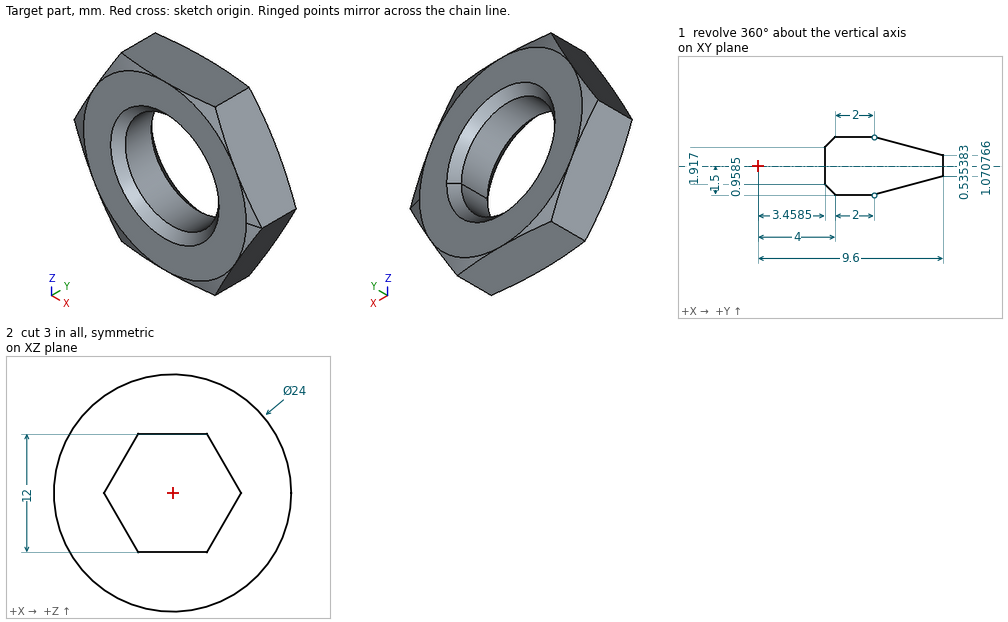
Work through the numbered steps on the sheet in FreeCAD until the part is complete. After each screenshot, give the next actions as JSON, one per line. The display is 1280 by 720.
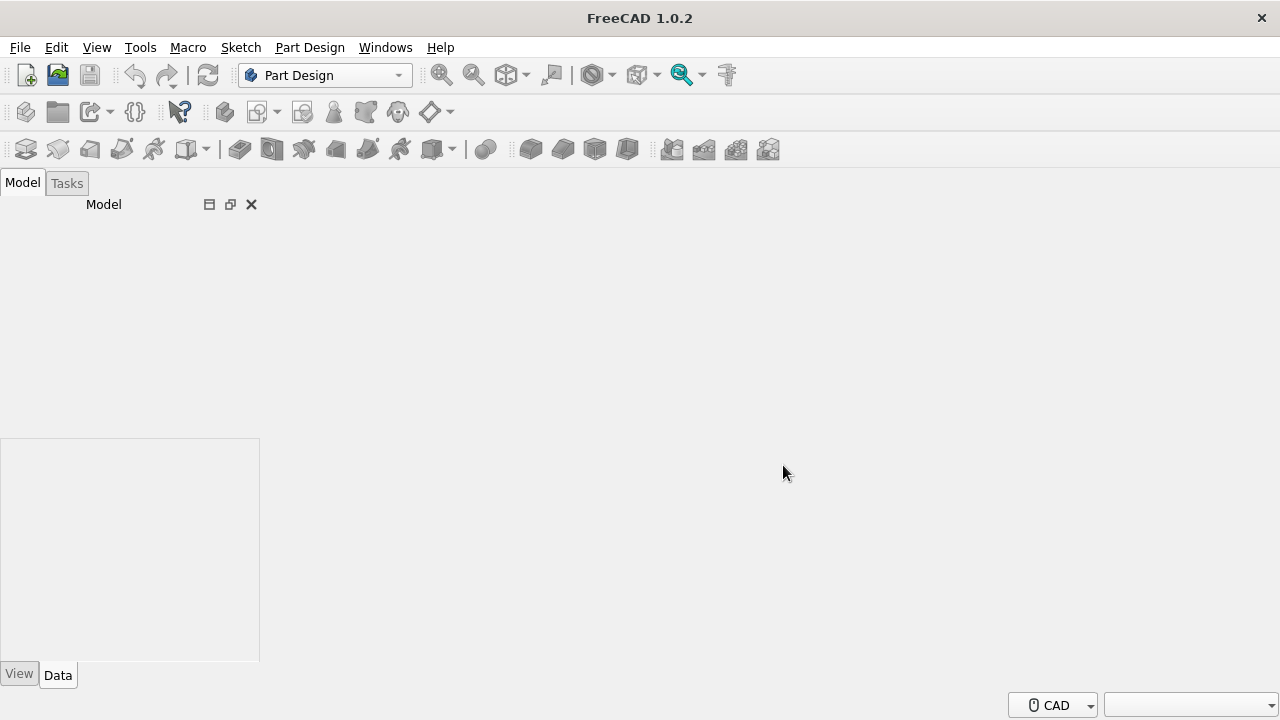
{"action": "left_click", "coordinate": [26, 76]}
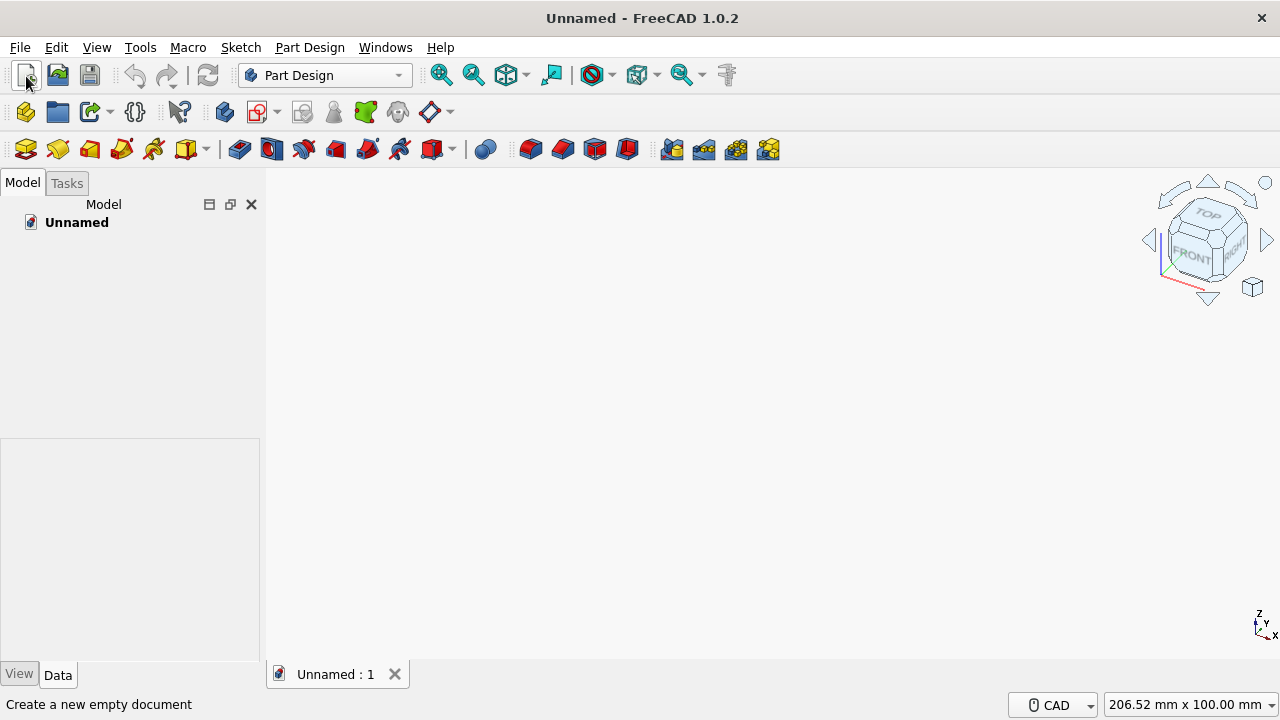
{"action": "left_click", "coordinate": [258, 112]}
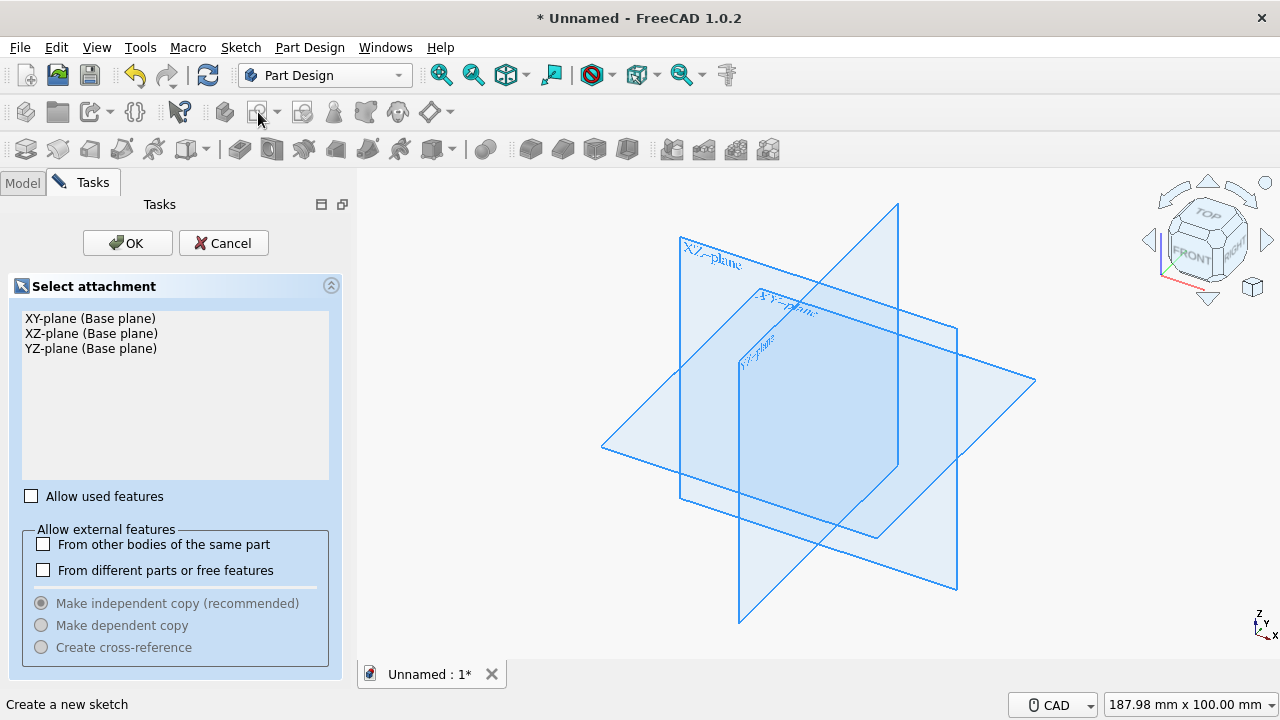
{"action": "left_click", "coordinate": [82, 318]}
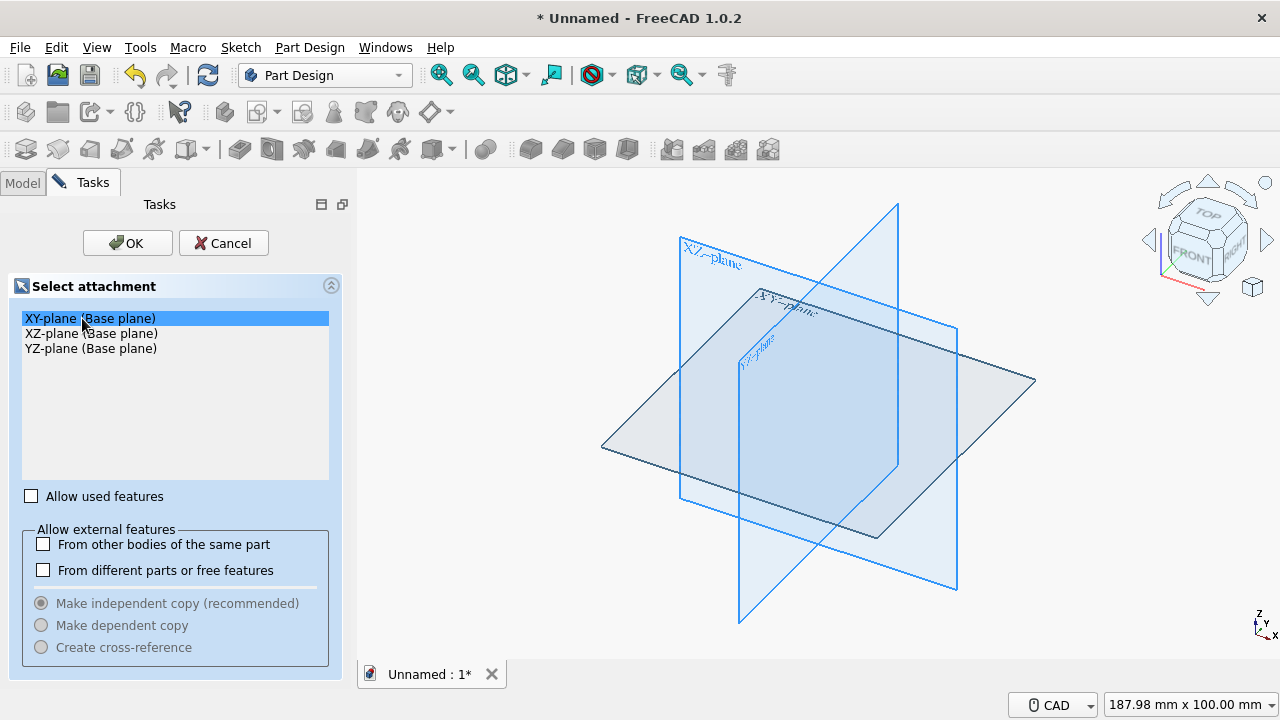
{"action": "left_click", "coordinate": [128, 243]}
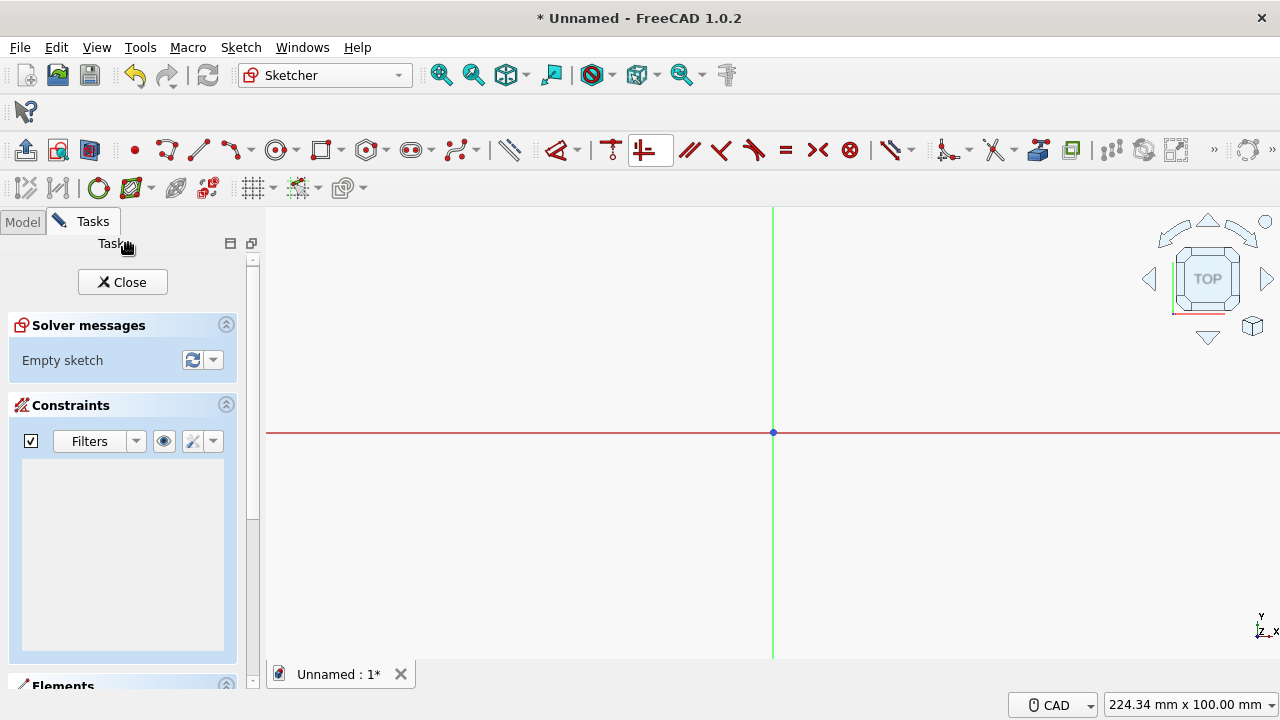
{"action": "scroll", "coordinate": [802, 433], "scroll_direction": "up", "scroll_amount": 13}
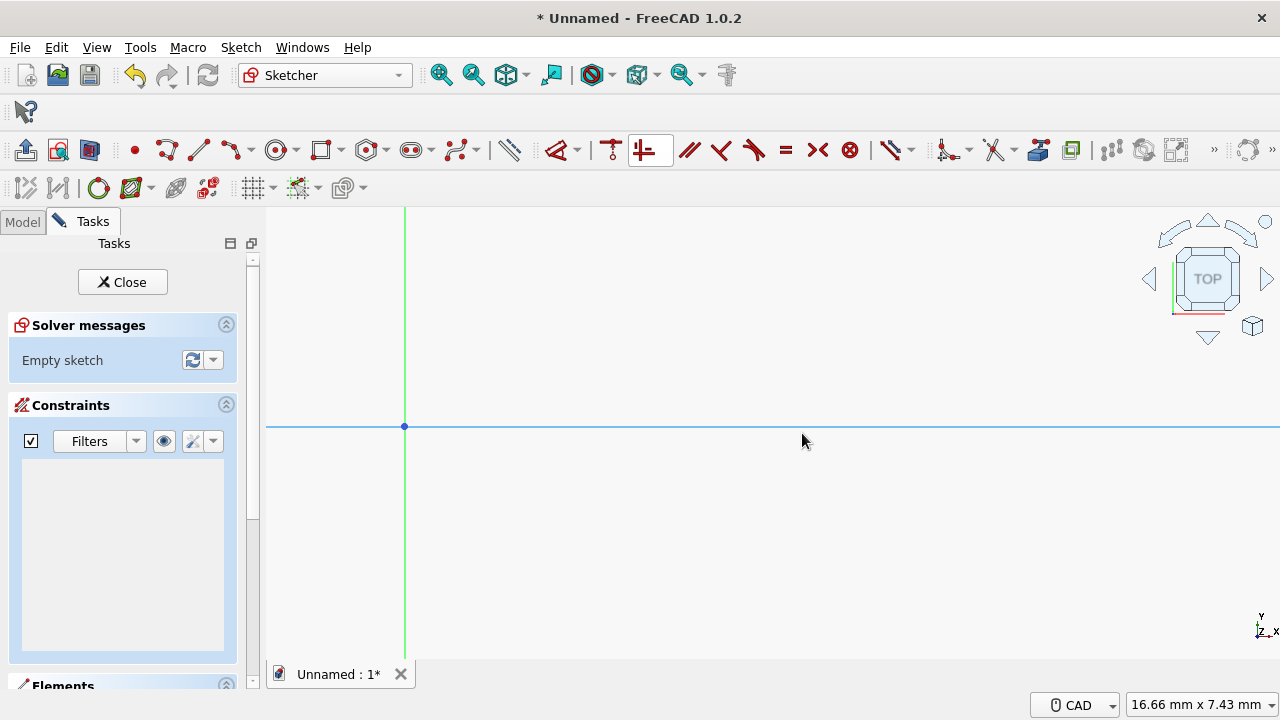
{"action": "left_click", "coordinate": [168, 150]}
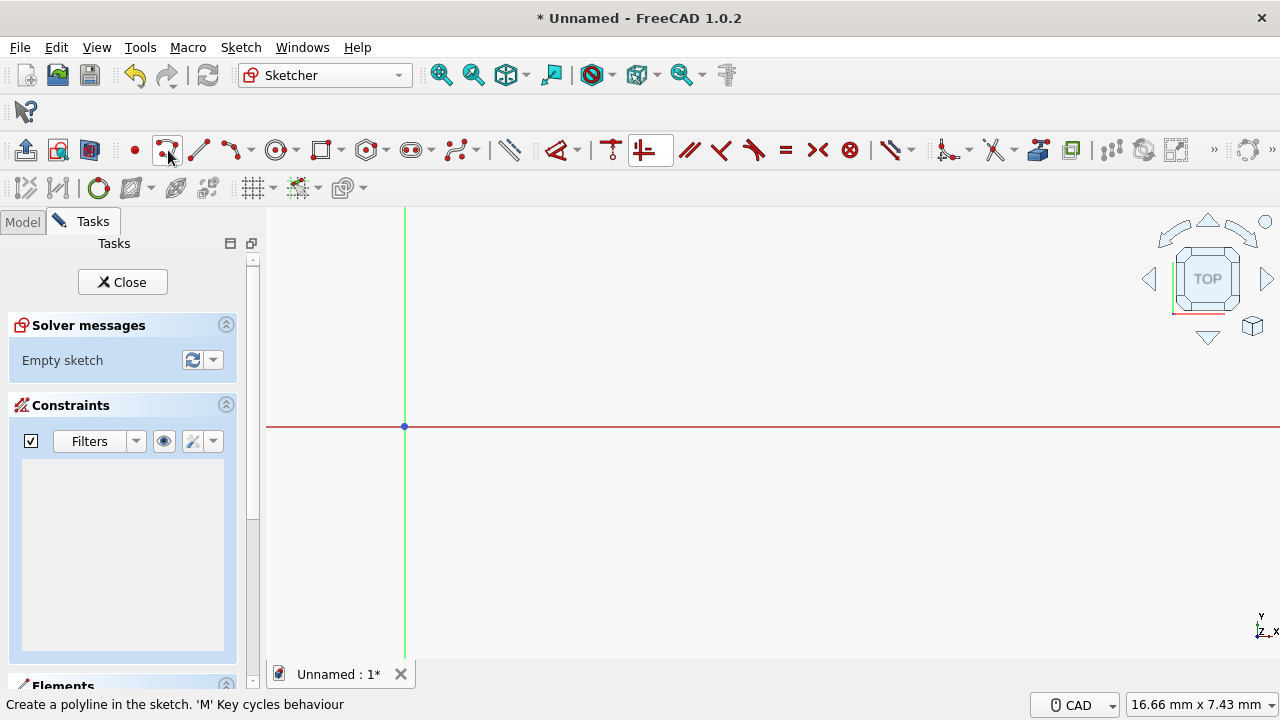
{"action": "left_click", "coordinate": [615, 485]}
{"action": "left_click", "coordinate": [648, 518]}
{"action": "left_click", "coordinate": [770, 518]}
{"action": "left_click", "coordinate": [989, 459]}
{"action": "left_click", "coordinate": [989, 394]}
{"action": "left_click", "coordinate": [770, 335]}
{"action": "left_click", "coordinate": [648, 335]}
{"action": "left_click", "coordinate": [615, 368]}
{"action": "left_click", "coordinate": [615, 486]}
{"action": "key", "text": "Escape"}
{"action": "key", "text": "Escape"}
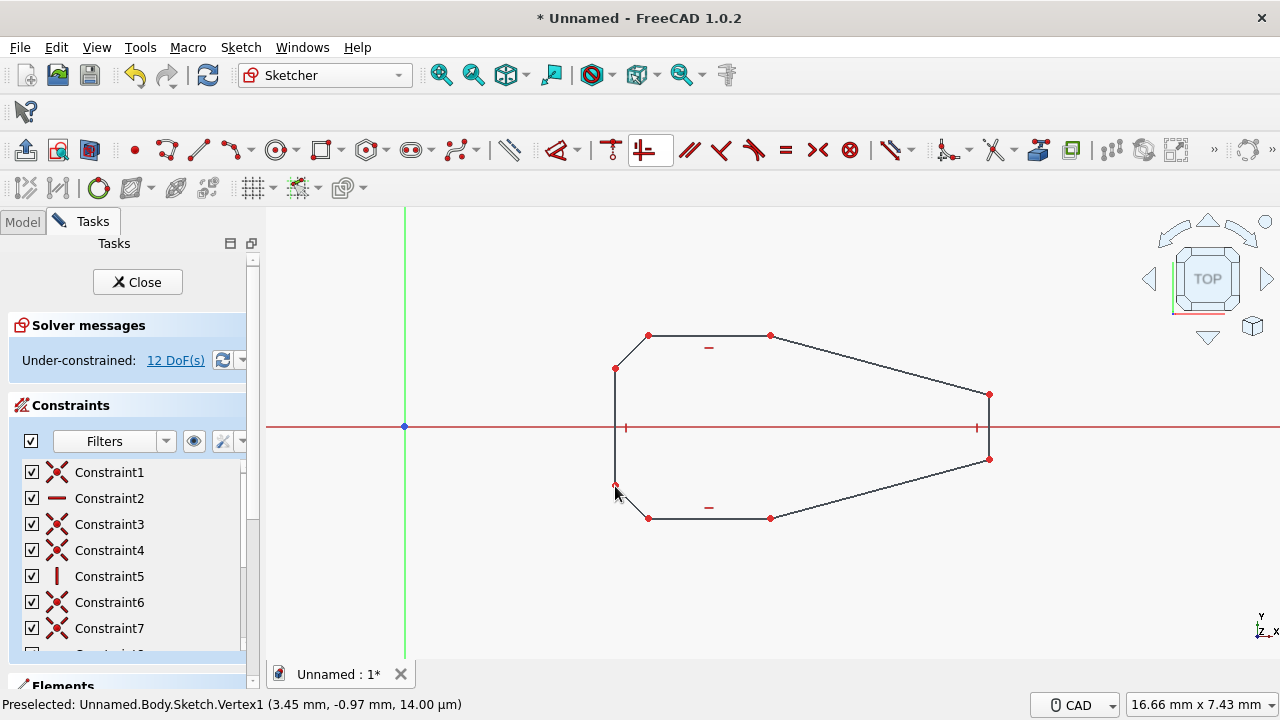
{"action": "left_click", "coordinate": [770, 519]}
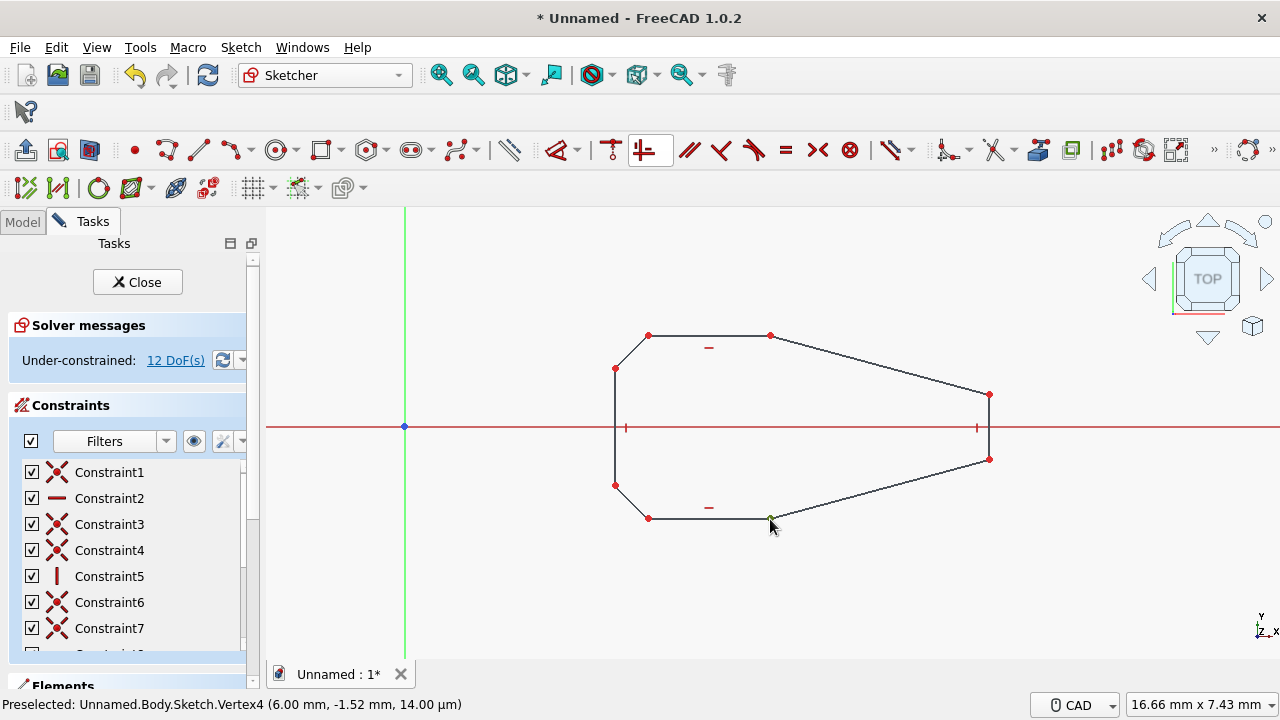
{"action": "left_click", "coordinate": [770, 336]}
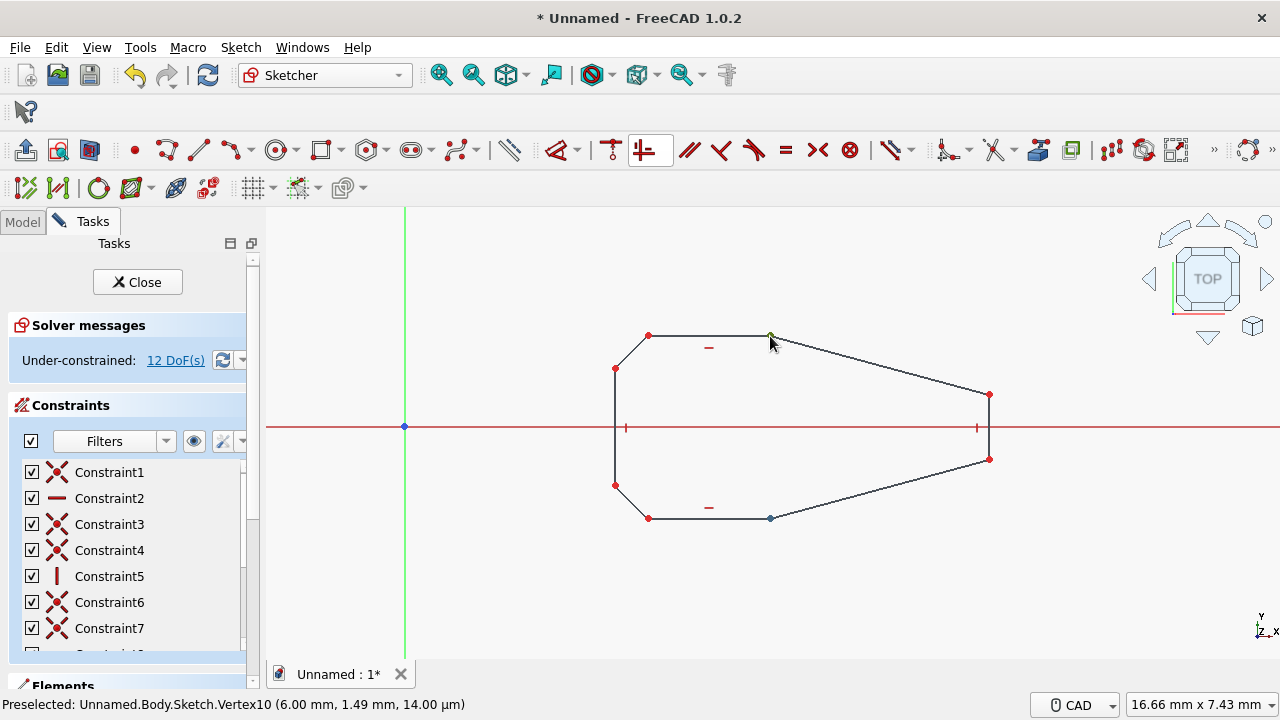
{"action": "left_click", "coordinate": [353, 427]}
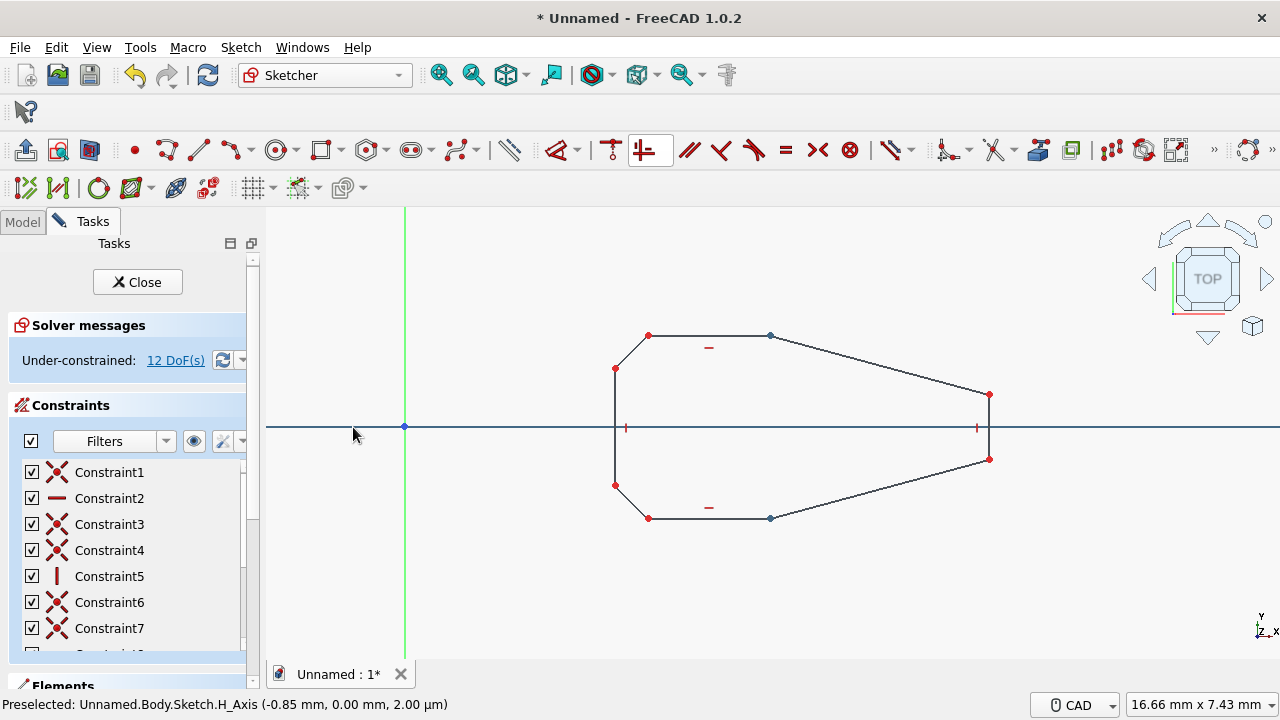
{"action": "left_click", "coordinate": [818, 150]}